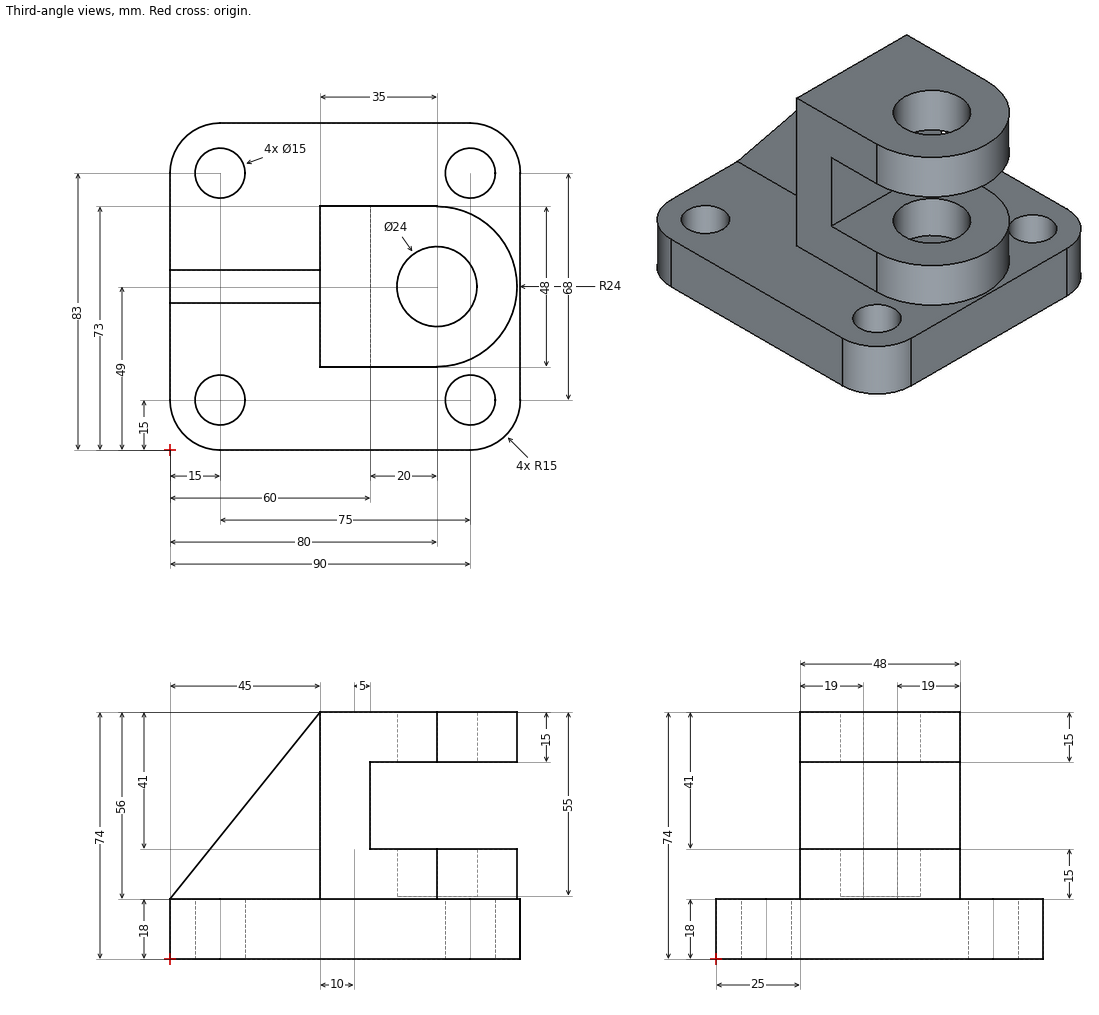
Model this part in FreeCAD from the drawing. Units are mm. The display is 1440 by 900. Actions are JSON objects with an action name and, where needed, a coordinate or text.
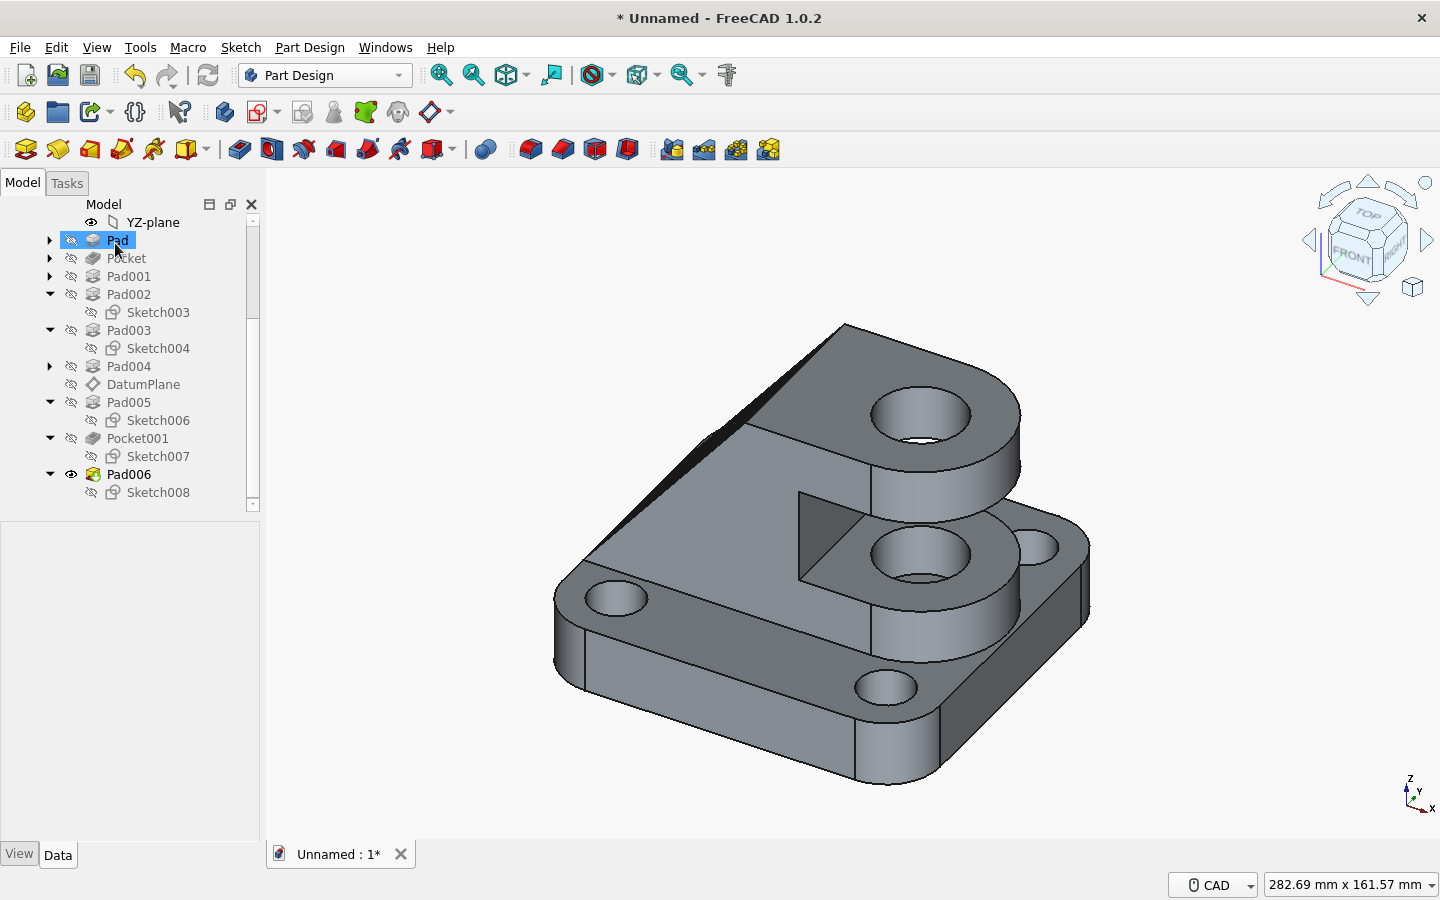
{"action": "left_click", "coordinate": [727, 538]}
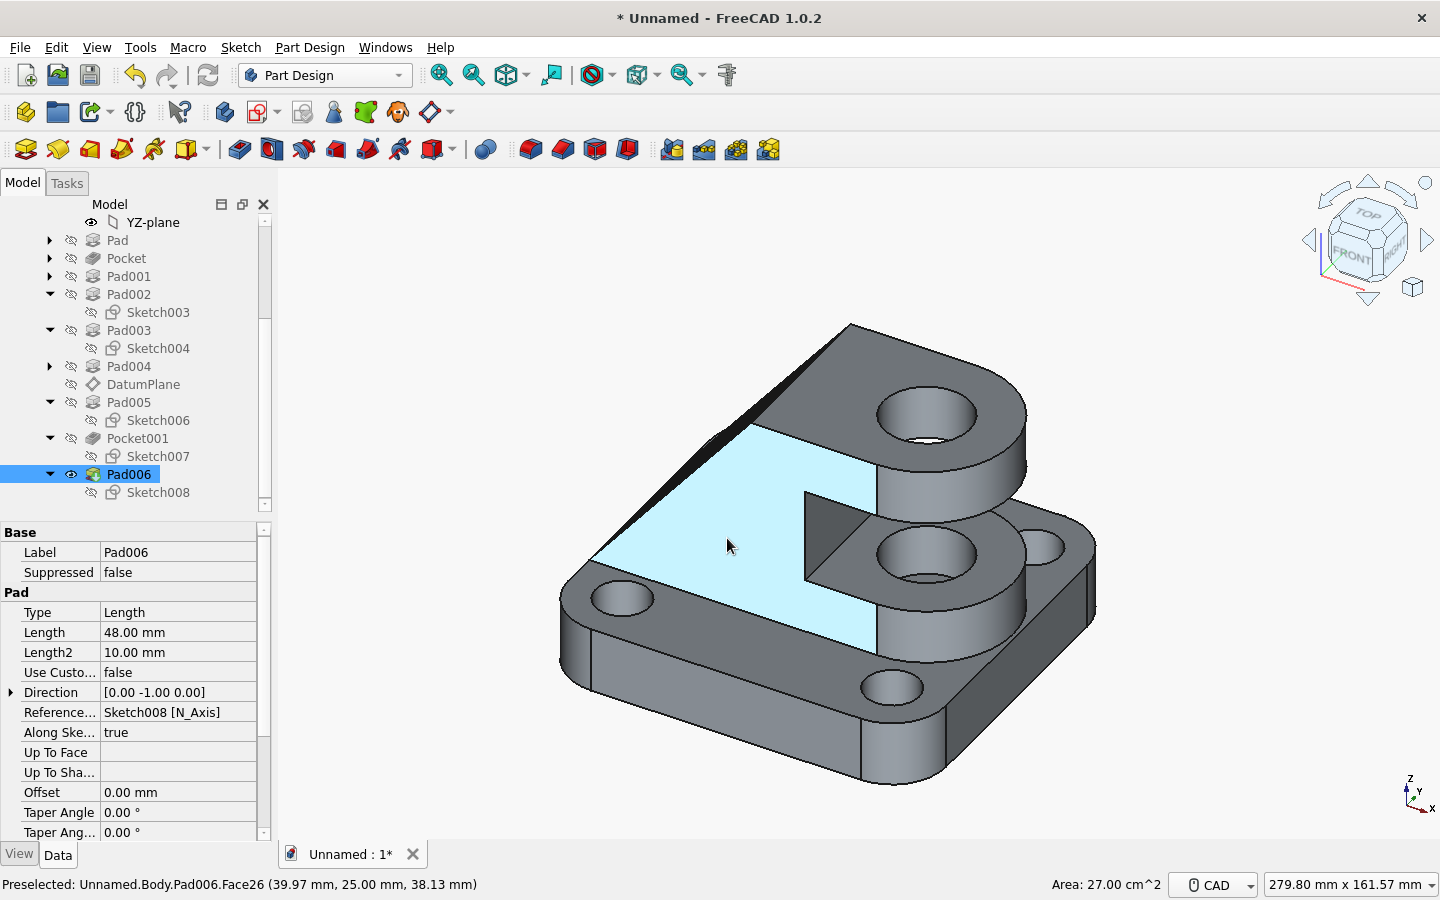
{"action": "left_click", "coordinate": [258, 112]}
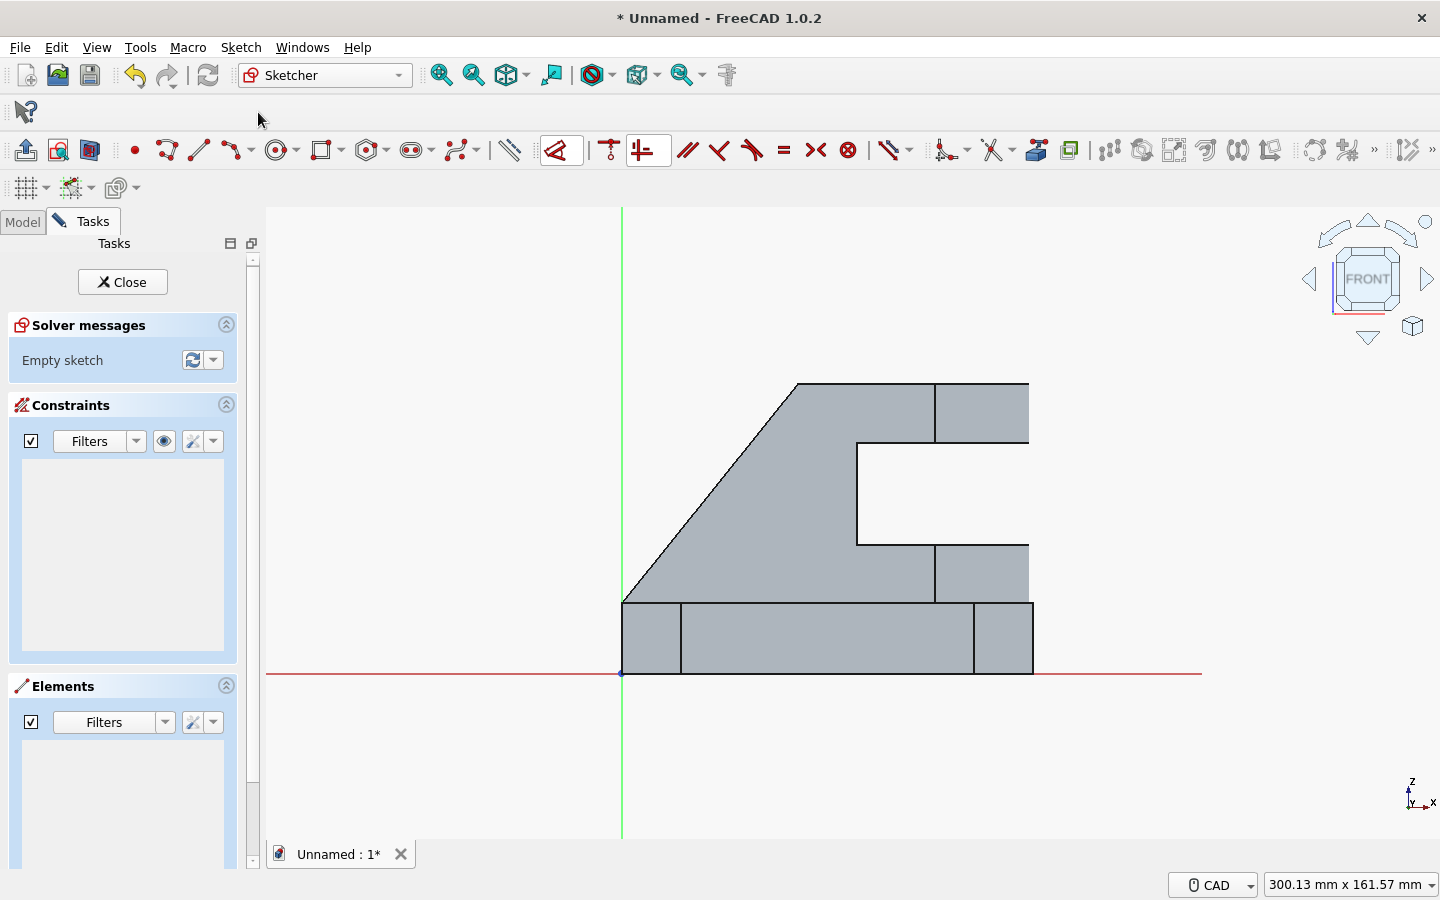
{"action": "left_click", "coordinate": [90, 150]}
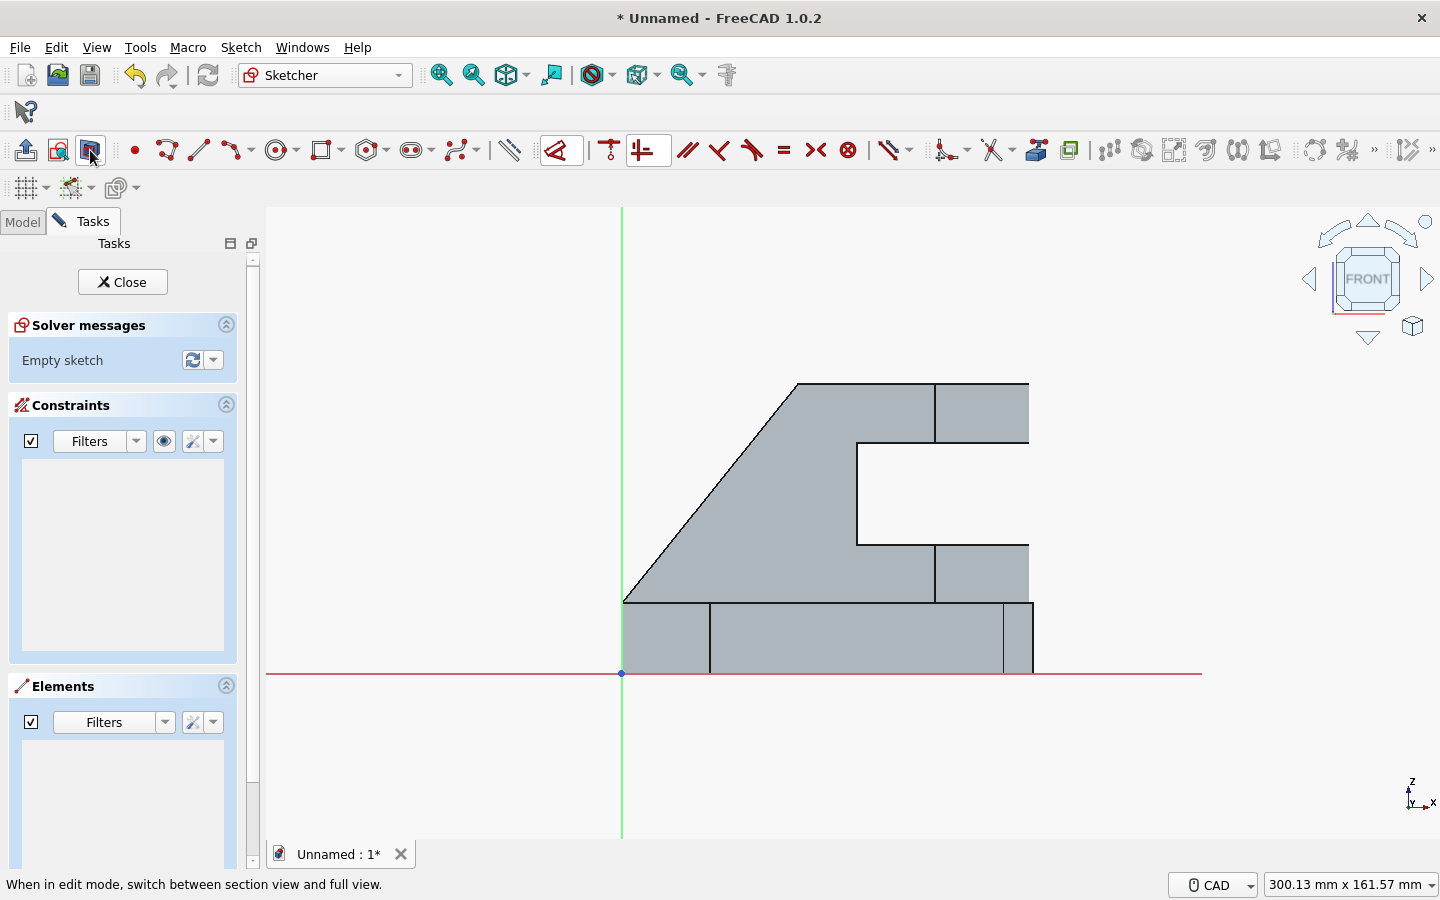
{"action": "scroll", "coordinate": [558, 541], "scroll_direction": "up", "scroll_amount": 2}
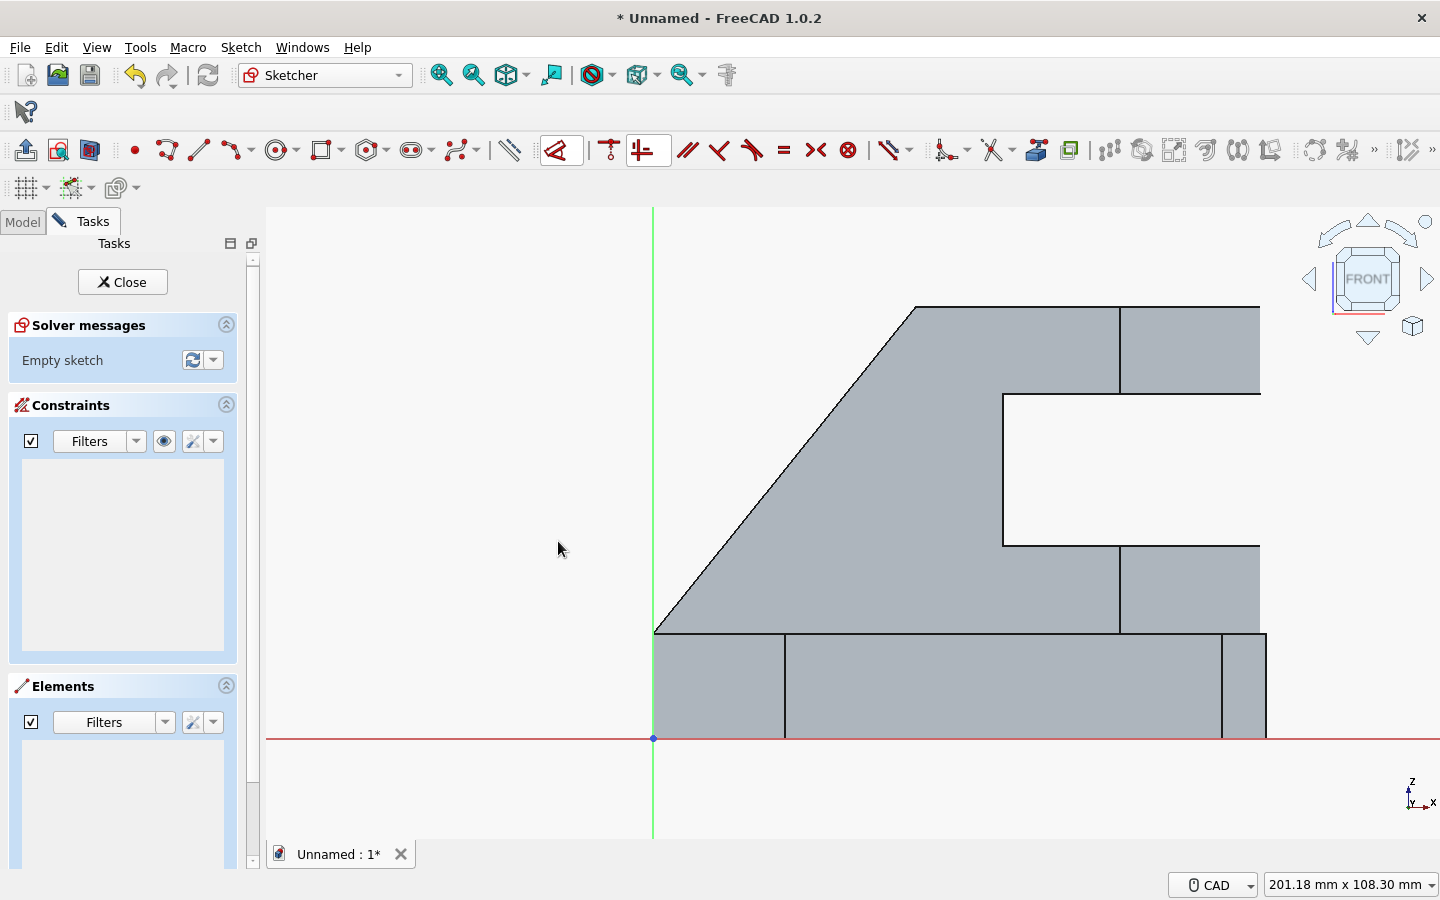
{"action": "left_click", "coordinate": [168, 150]}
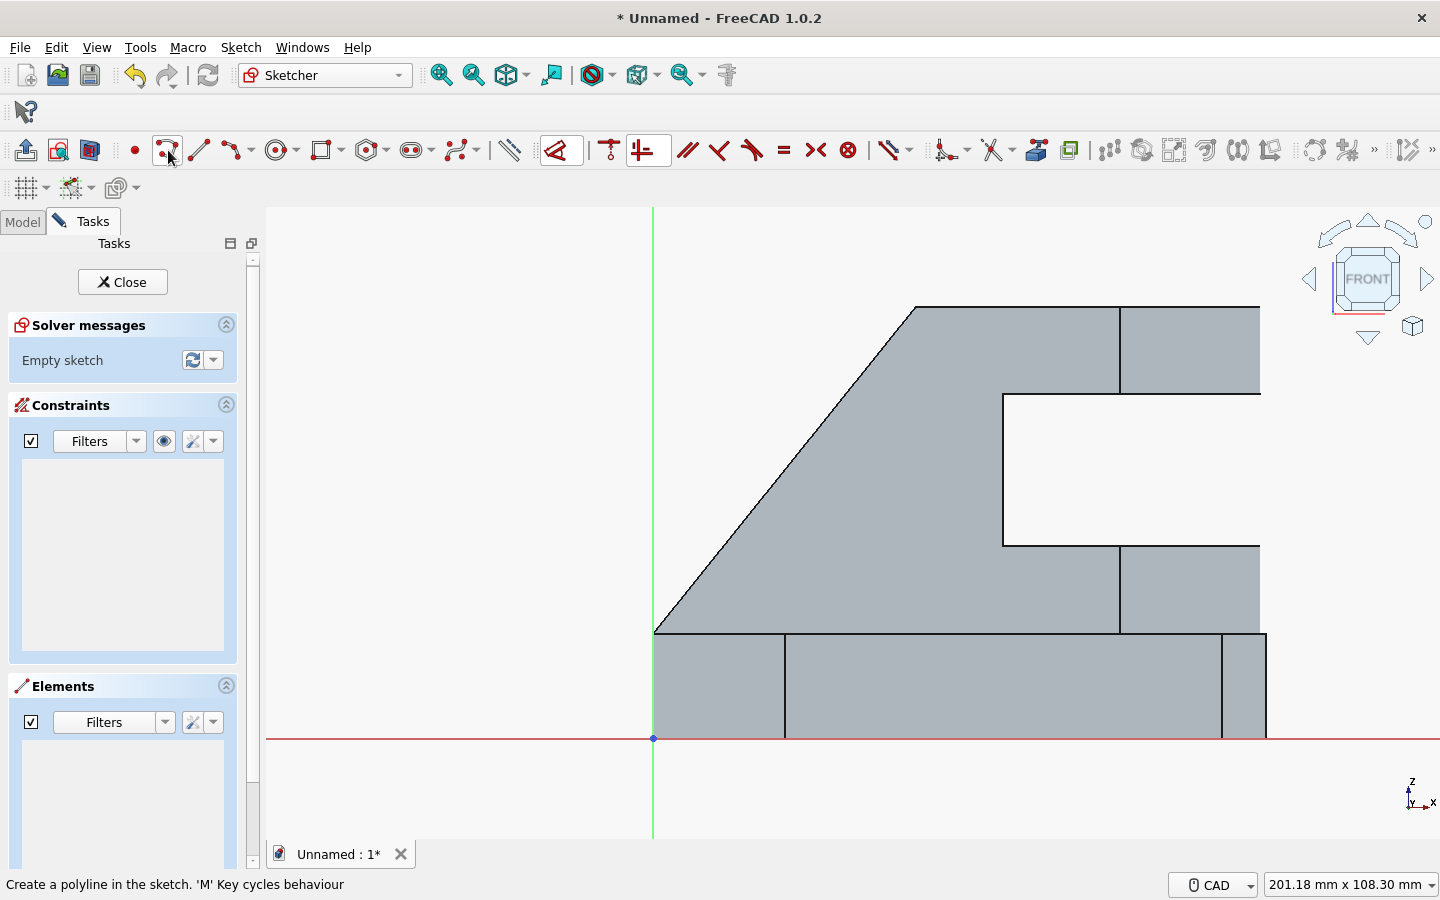
{"action": "left_click", "coordinate": [653, 634]}
{"action": "left_click", "coordinate": [916, 634]}
{"action": "left_click", "coordinate": [916, 307]}
{"action": "left_click", "coordinate": [653, 635]}
{"action": "key", "text": "Escape"}
{"action": "key", "text": "Escape"}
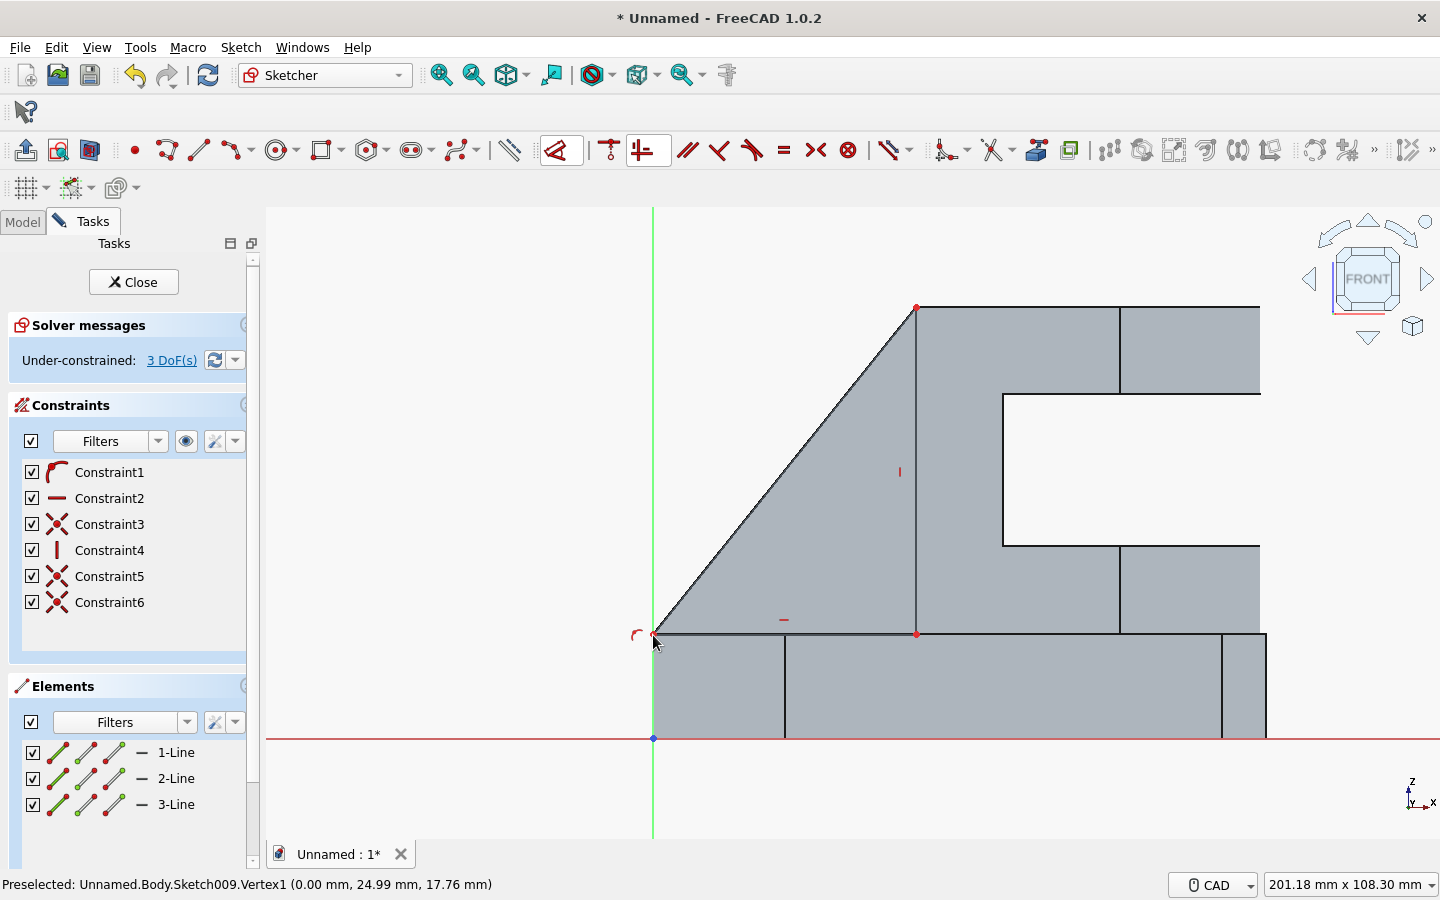
{"action": "left_click", "coordinate": [732, 635]}